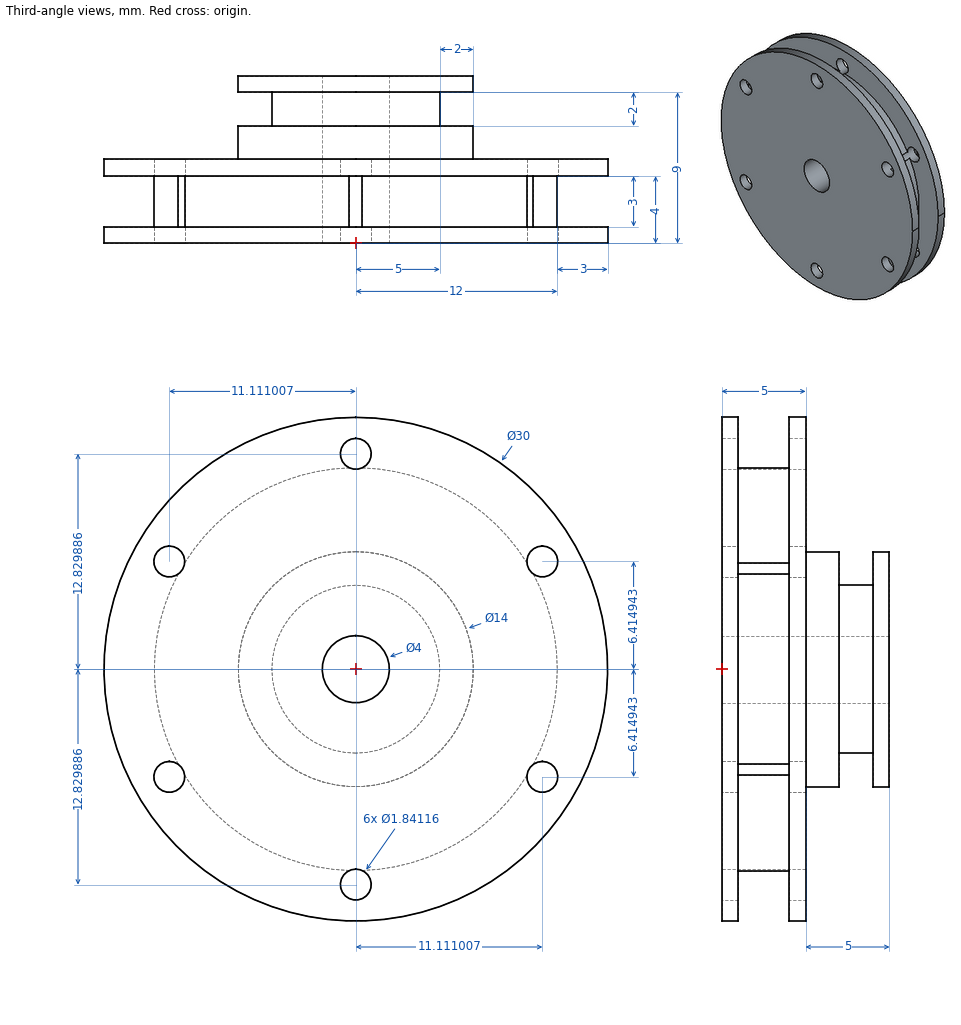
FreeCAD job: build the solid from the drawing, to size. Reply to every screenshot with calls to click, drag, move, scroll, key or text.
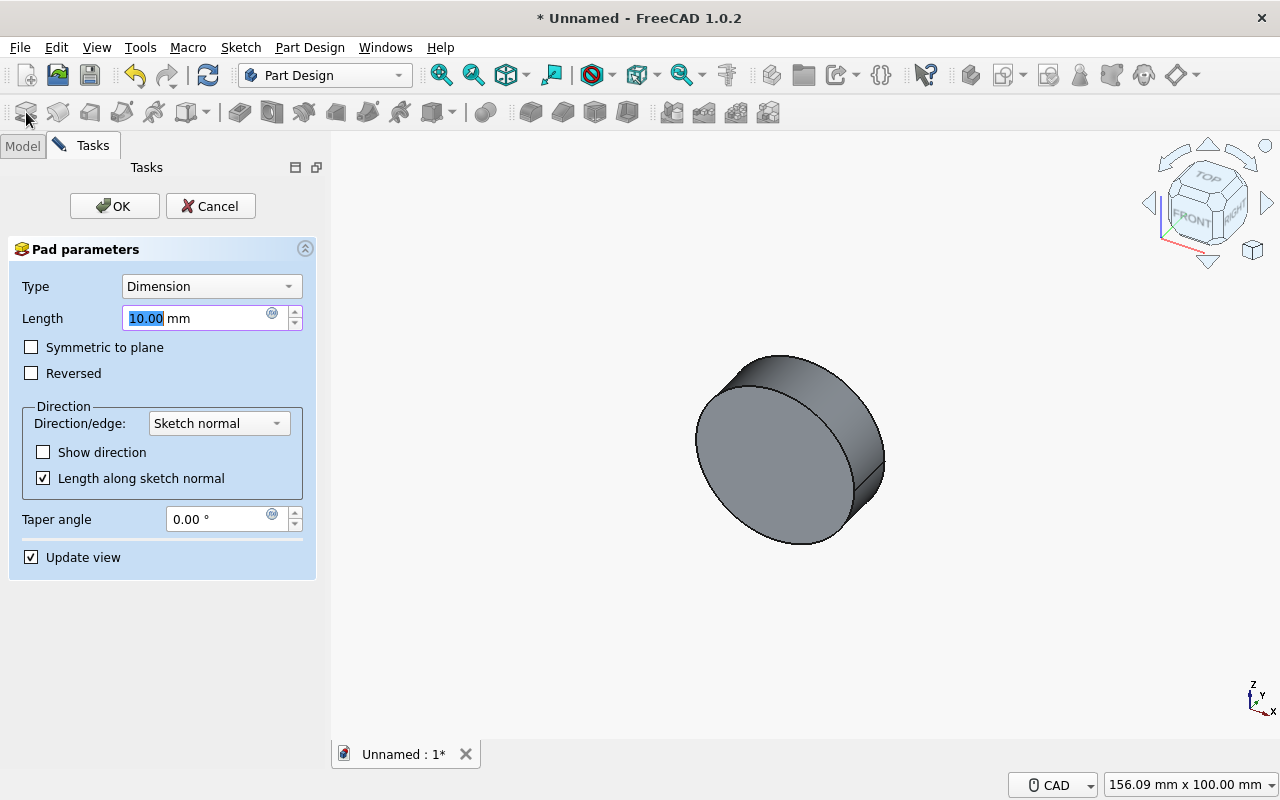
text(5)
key(Tab)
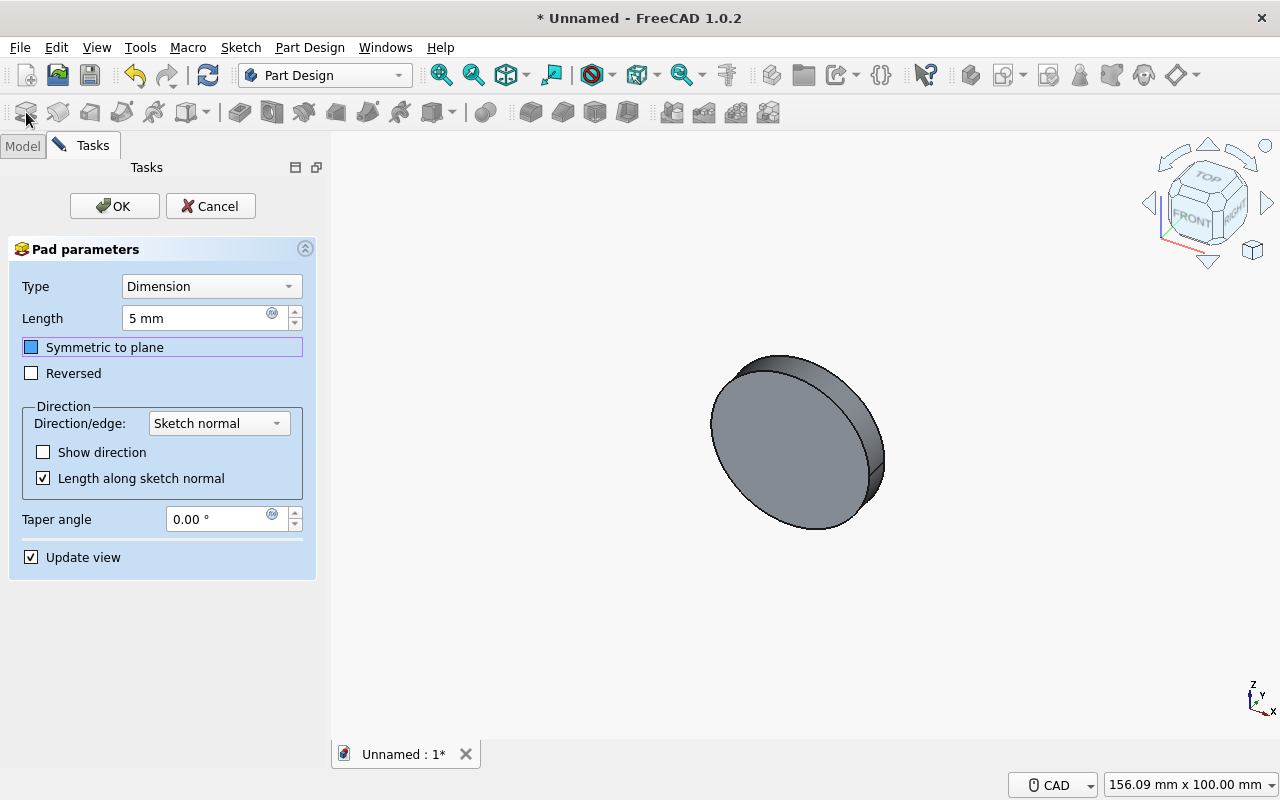
click(30, 373)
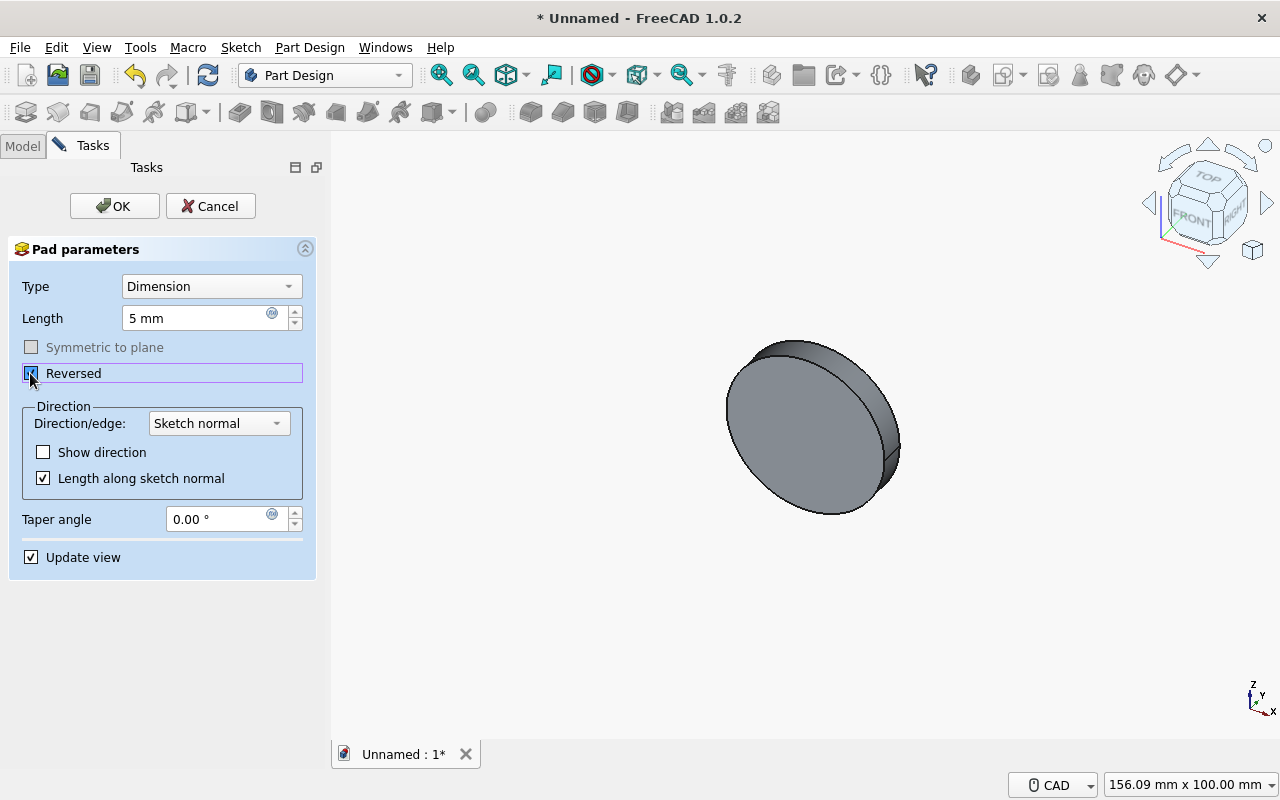
click(115, 206)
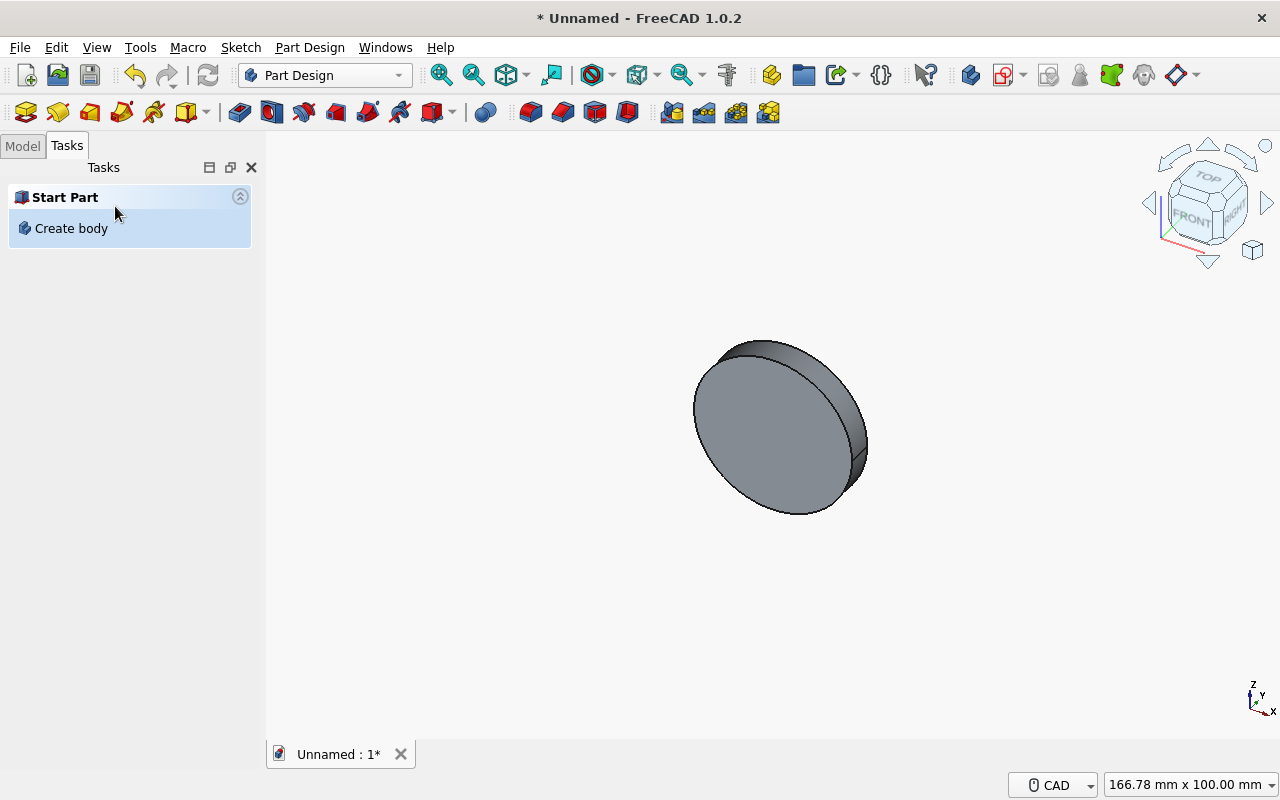
click(442, 76)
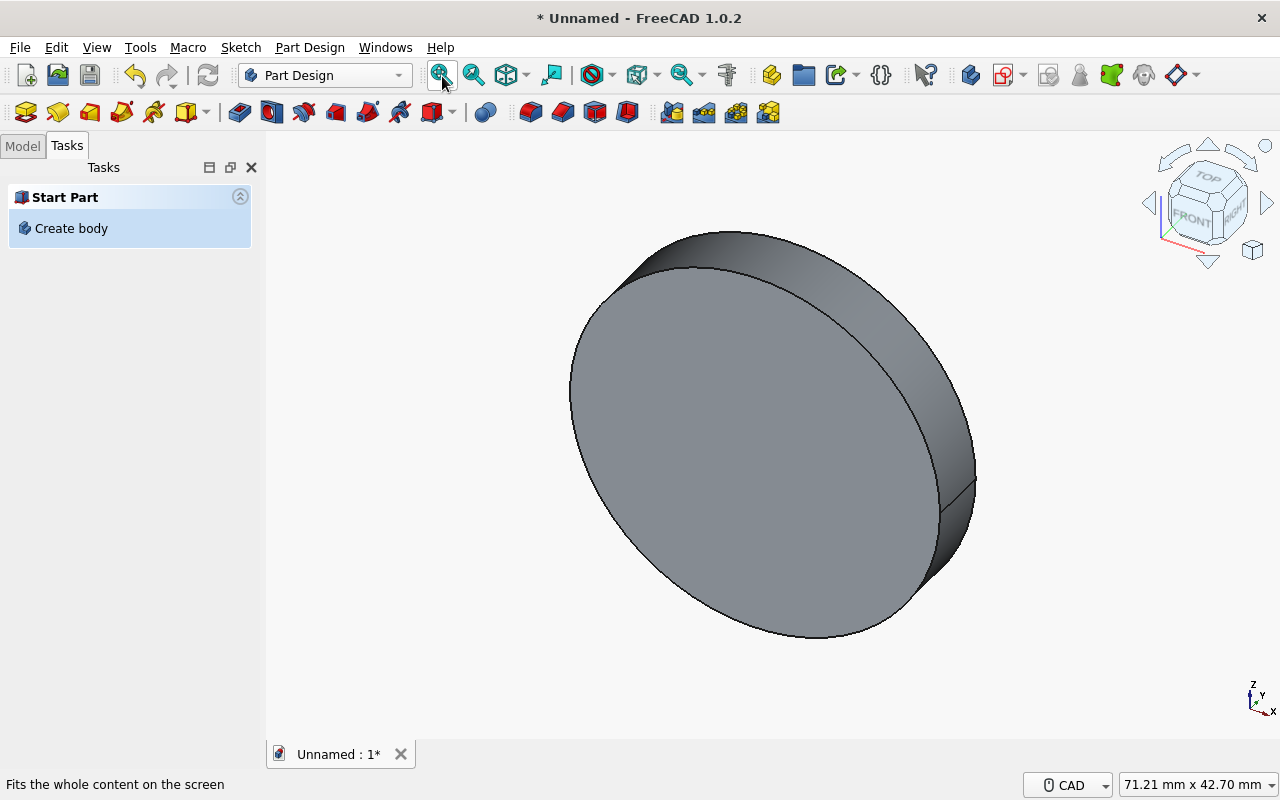
click(1004, 76)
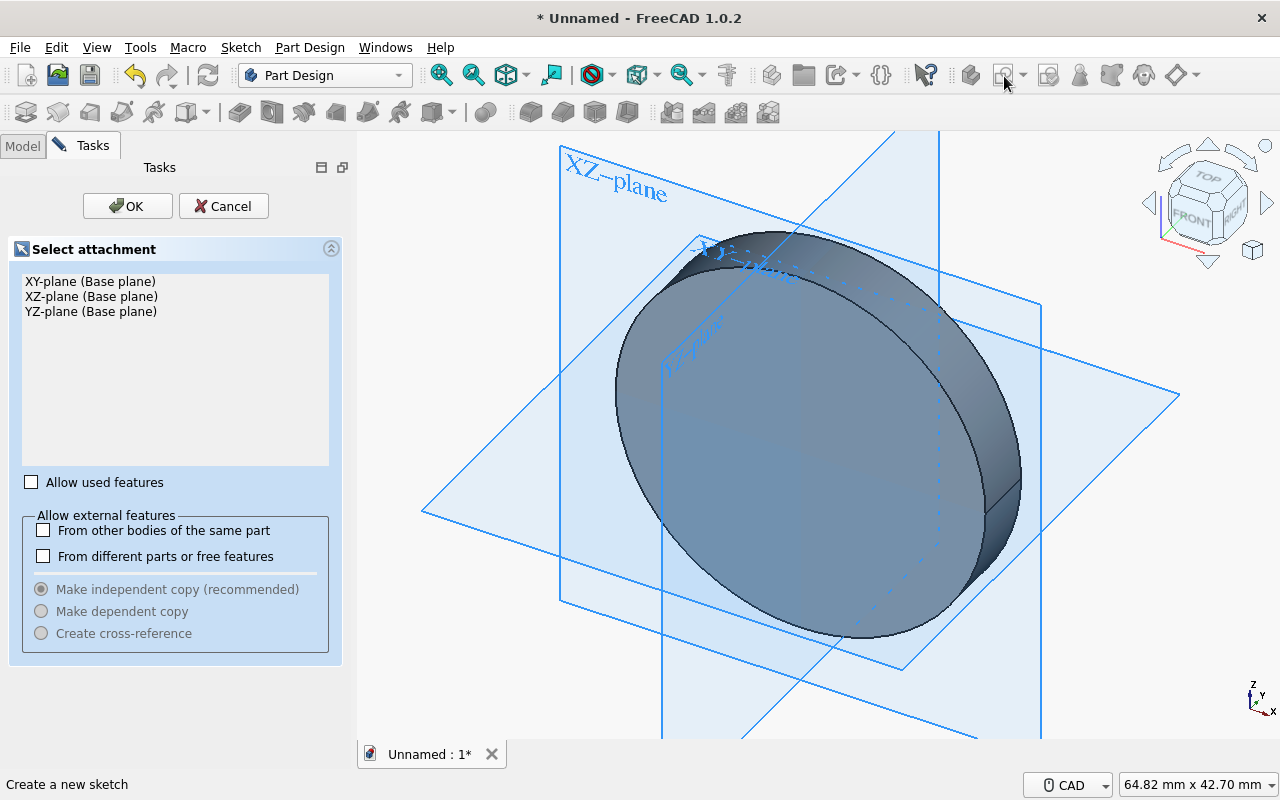
click(82, 282)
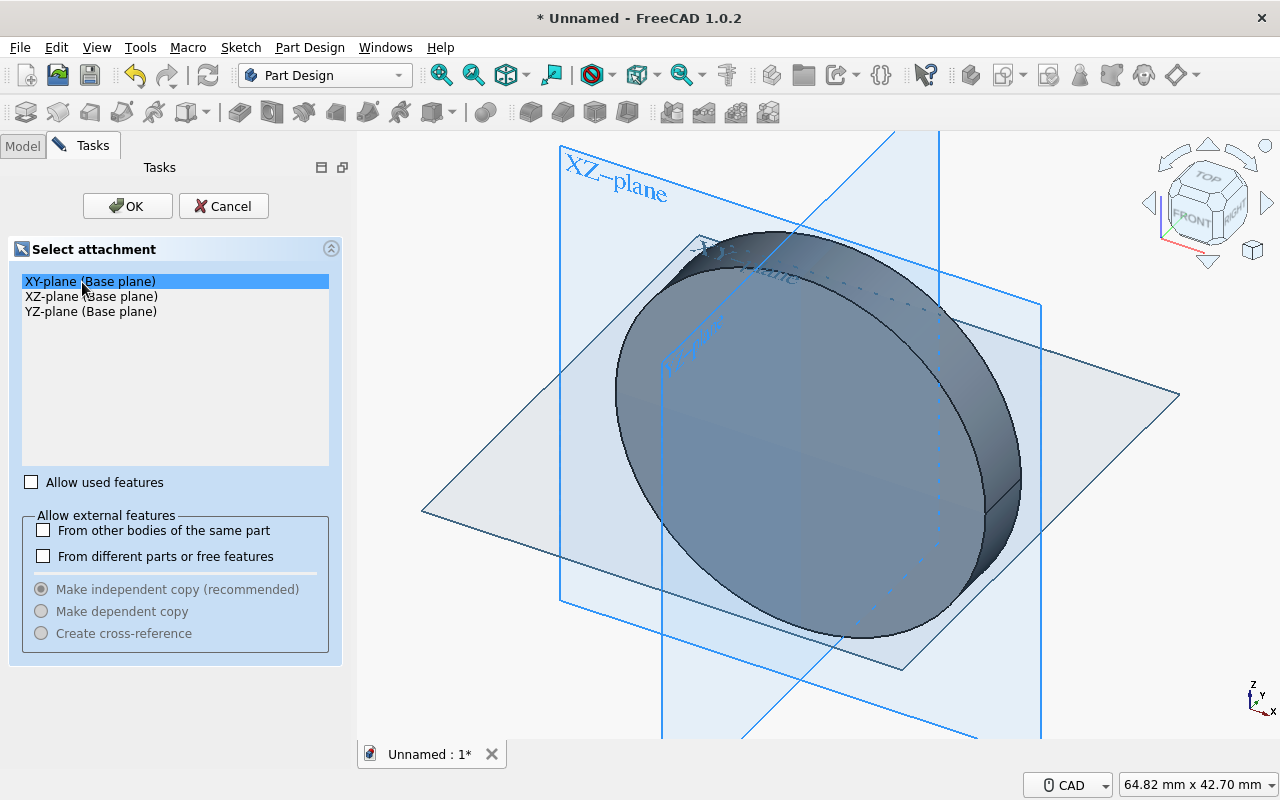
click(128, 206)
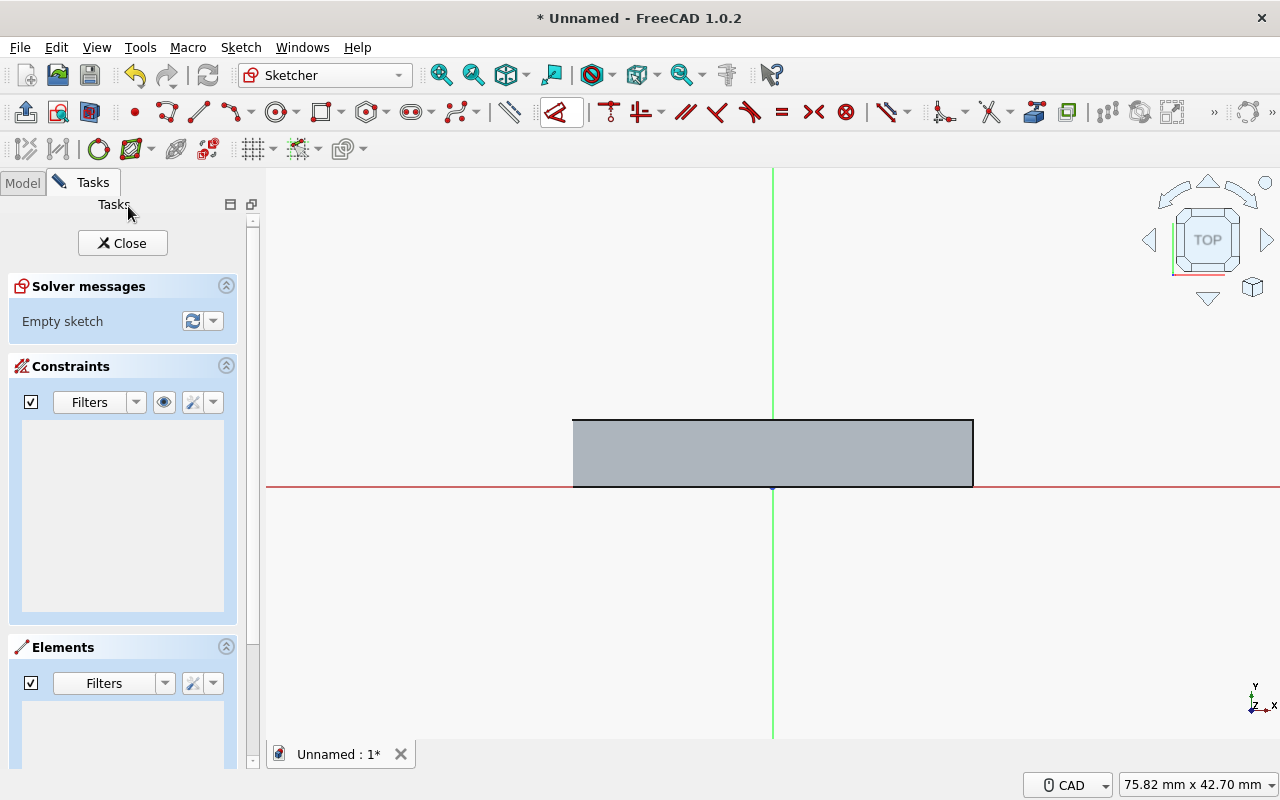
click(90, 112)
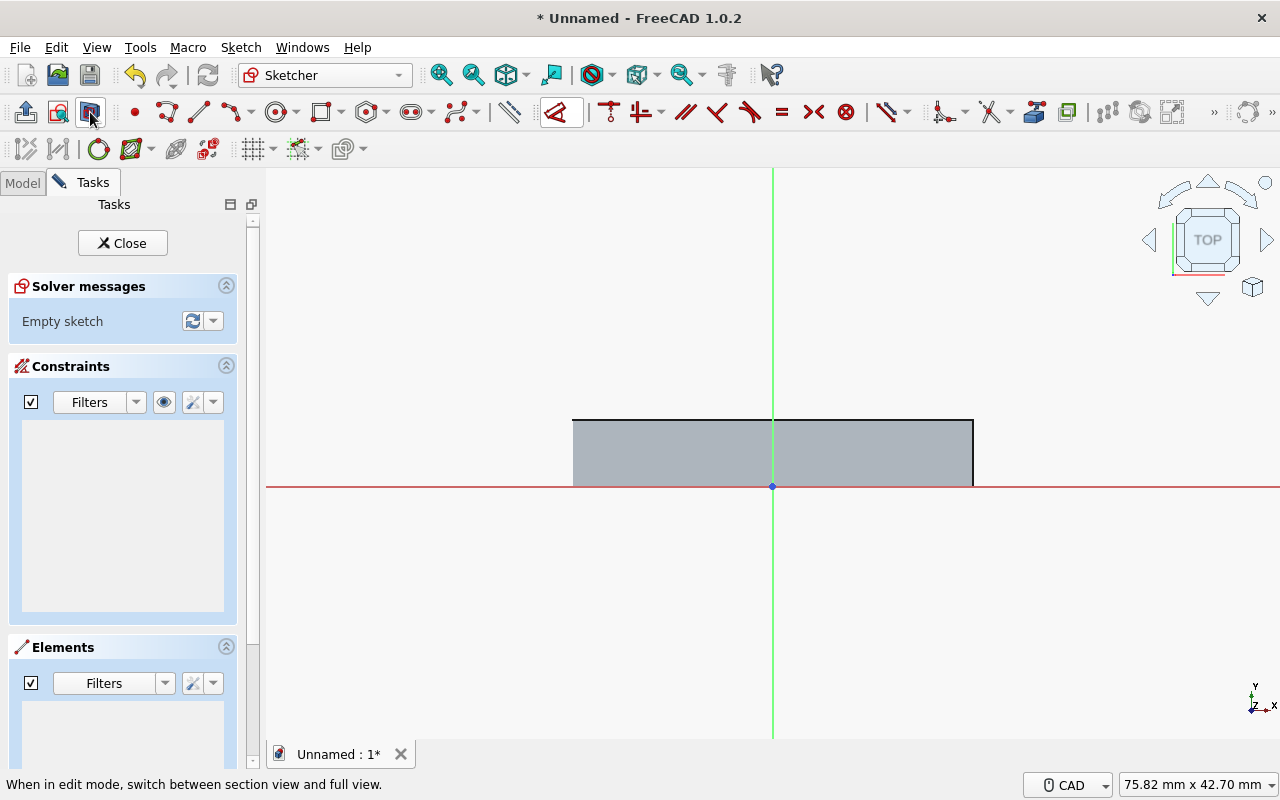
scroll(984, 454, up, 11)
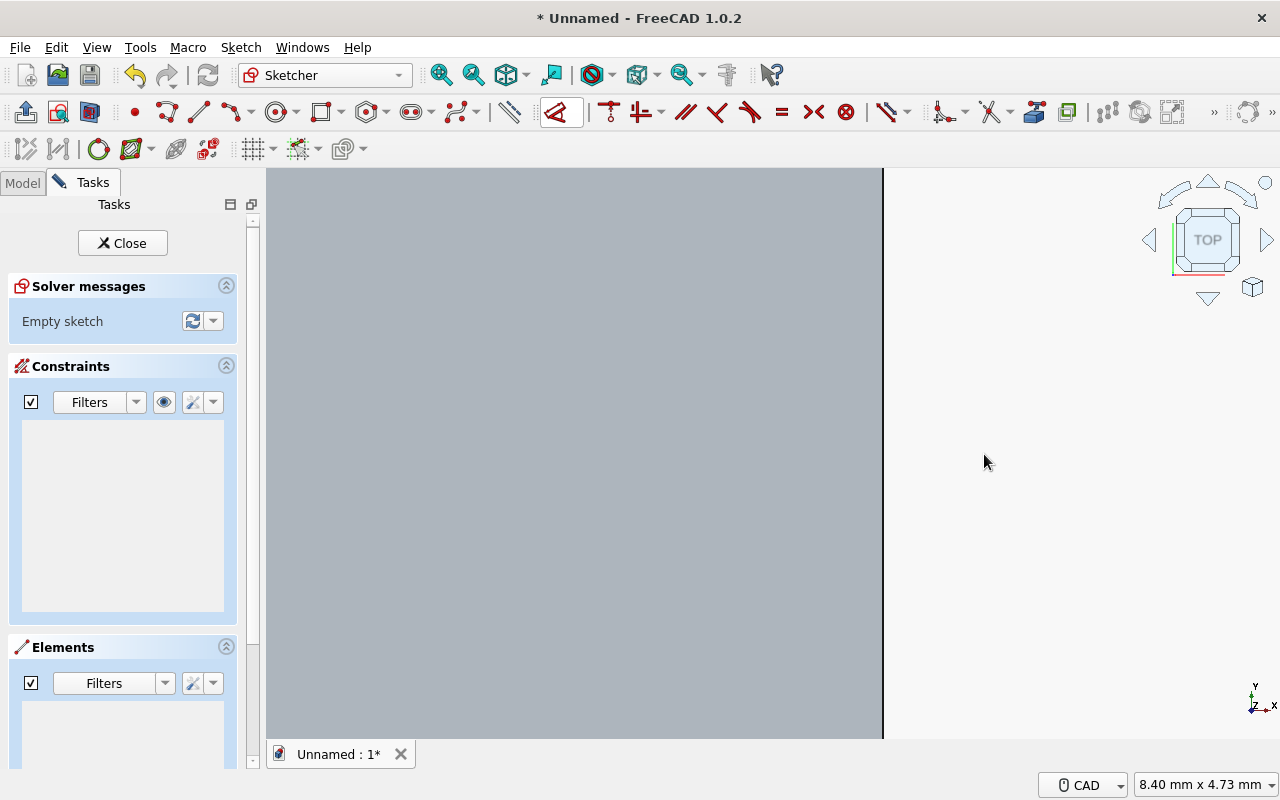
click(322, 112)